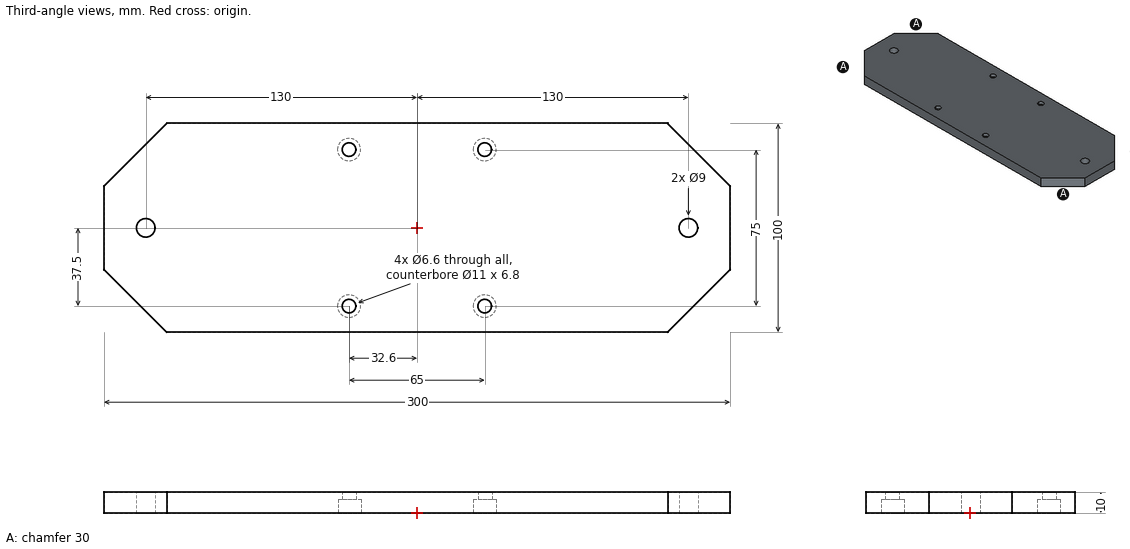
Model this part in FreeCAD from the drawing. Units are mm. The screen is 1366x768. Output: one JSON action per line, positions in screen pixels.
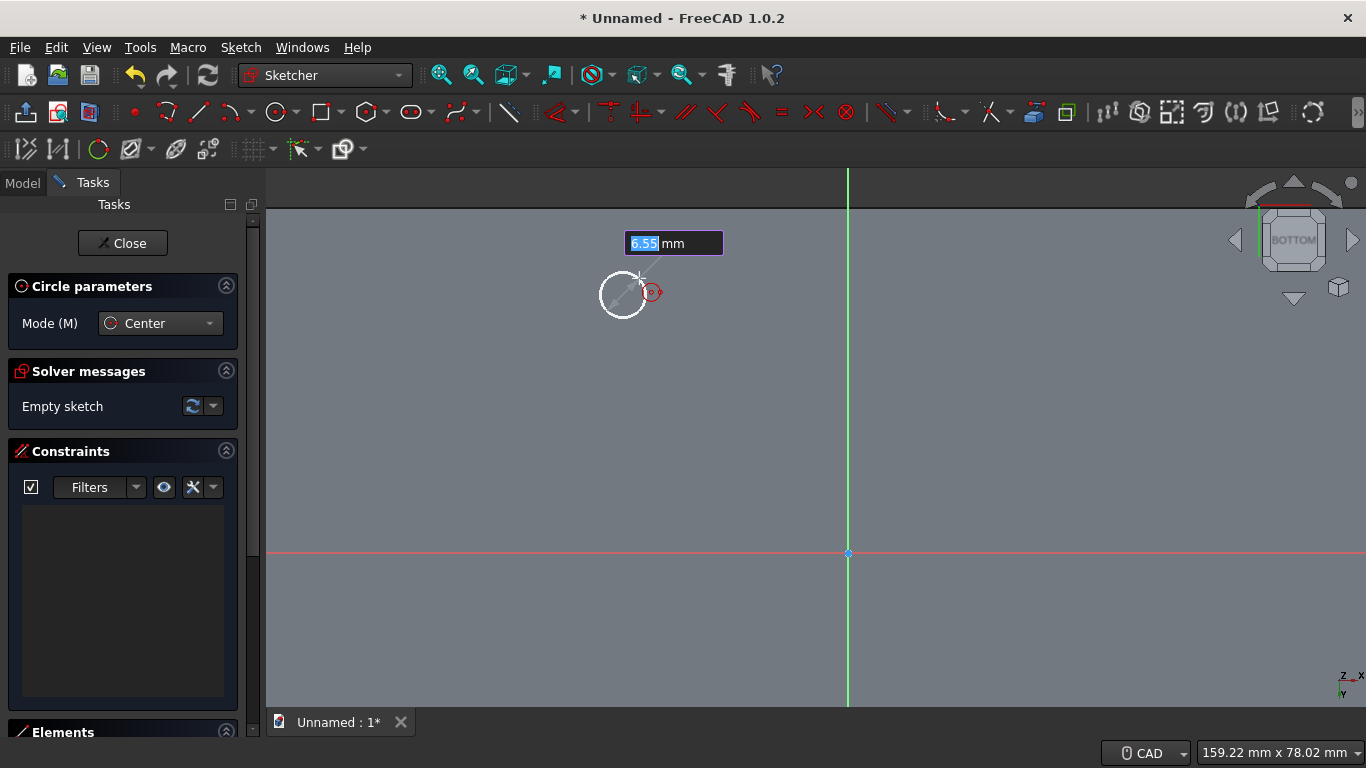
{"action": "type", "text": "6.6"}
{"action": "key", "text": "Return"}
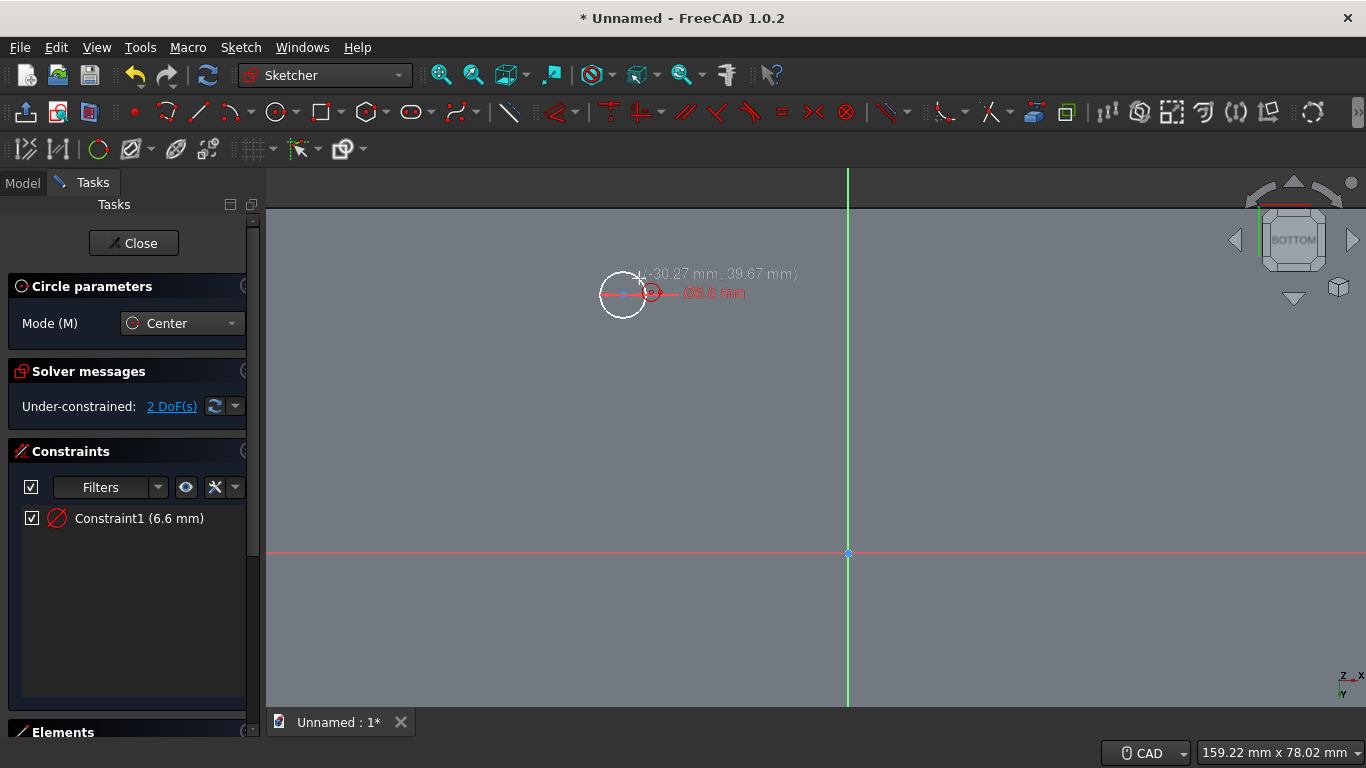
{"action": "left_click", "coordinate": [1072, 294]}
{"action": "mouse_move", "coordinate": [1088, 278]}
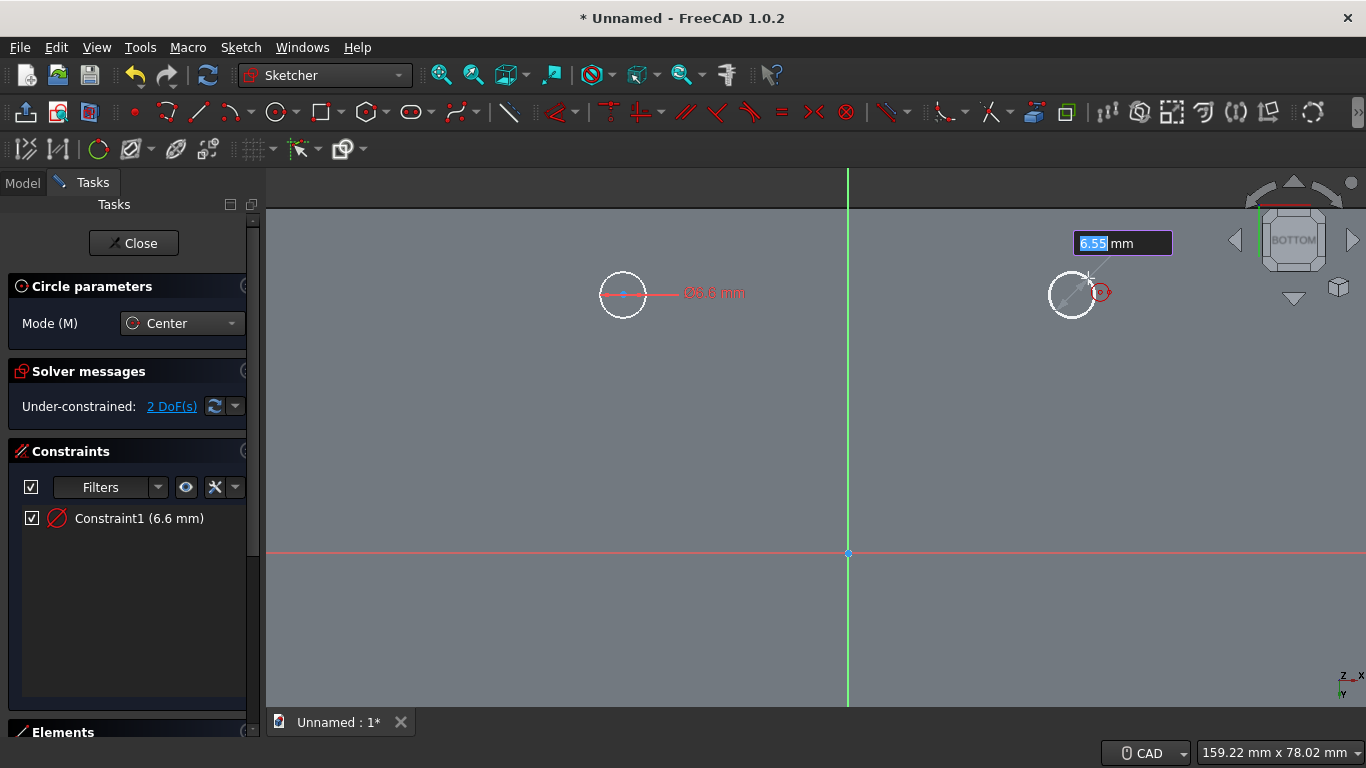
{"action": "type", "text": "6.6"}
{"action": "key", "text": "Return"}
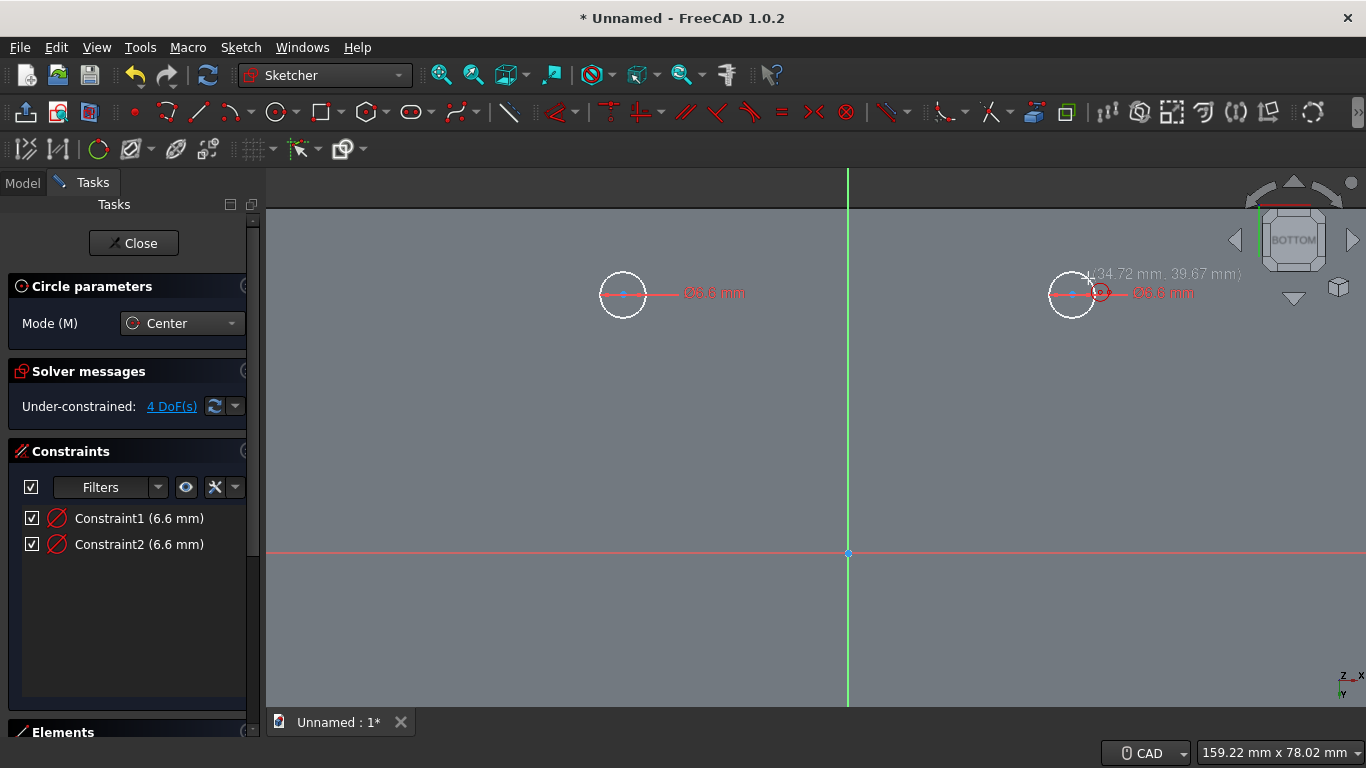
{"action": "scroll", "coordinate": [626, 297], "scroll_direction": "down", "scroll_amount": 3}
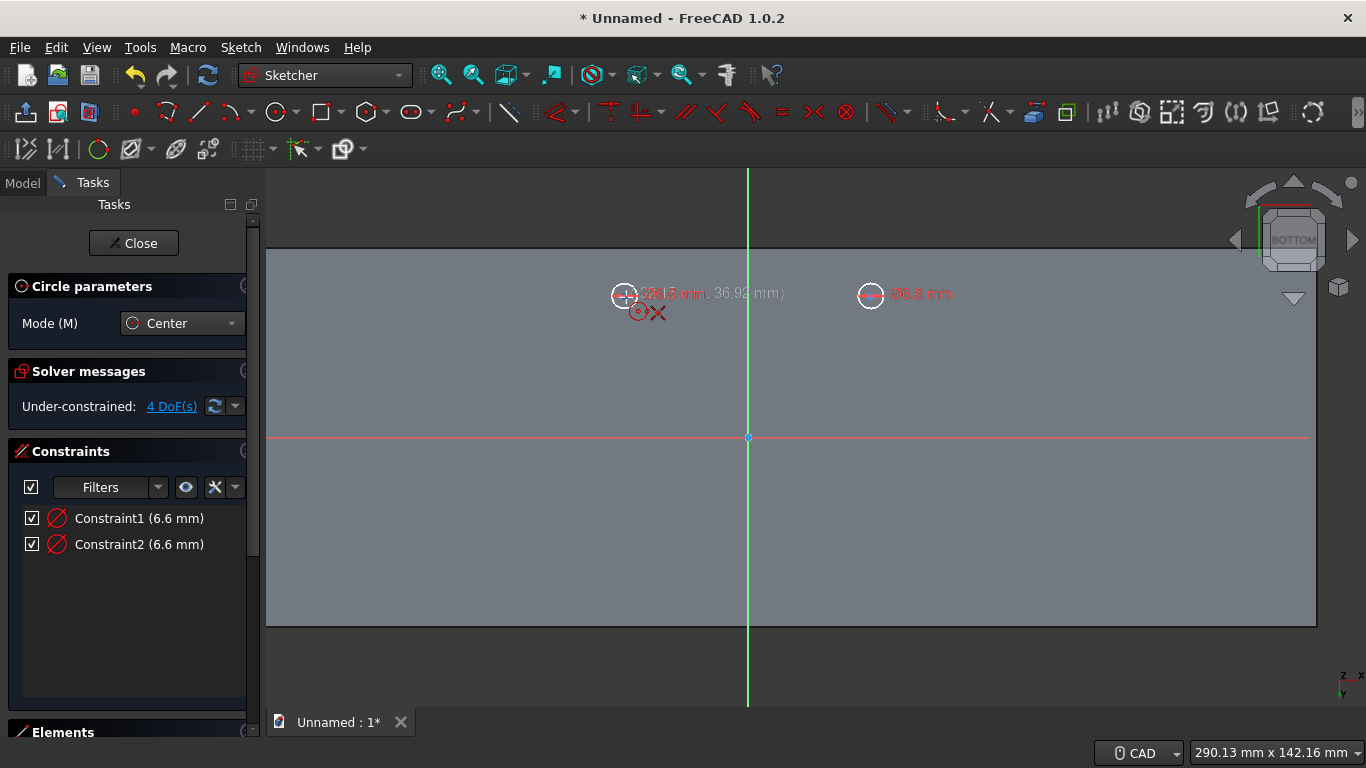
{"action": "scroll", "coordinate": [871, 580], "scroll_direction": "up", "scroll_amount": 3}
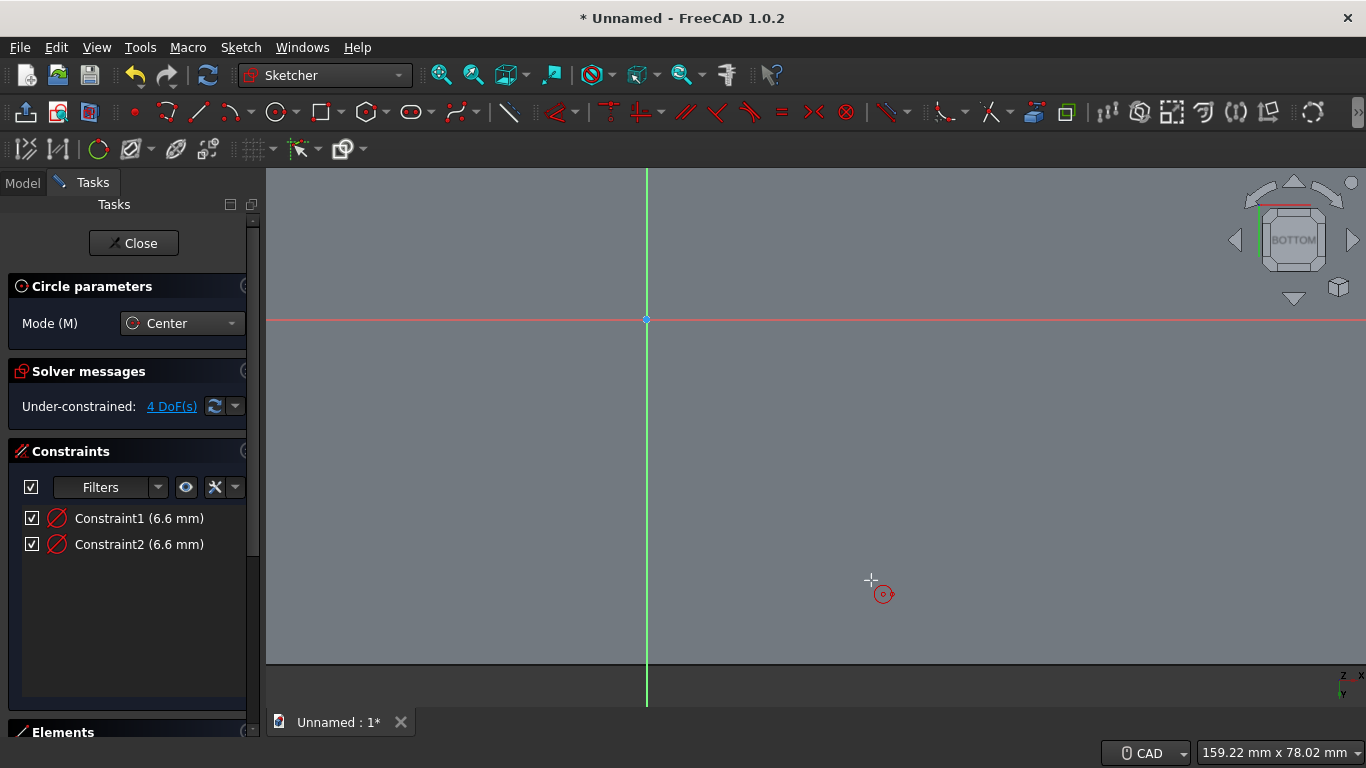
{"action": "left_click", "coordinate": [870, 579]}
{"action": "mouse_move", "coordinate": [886, 563]}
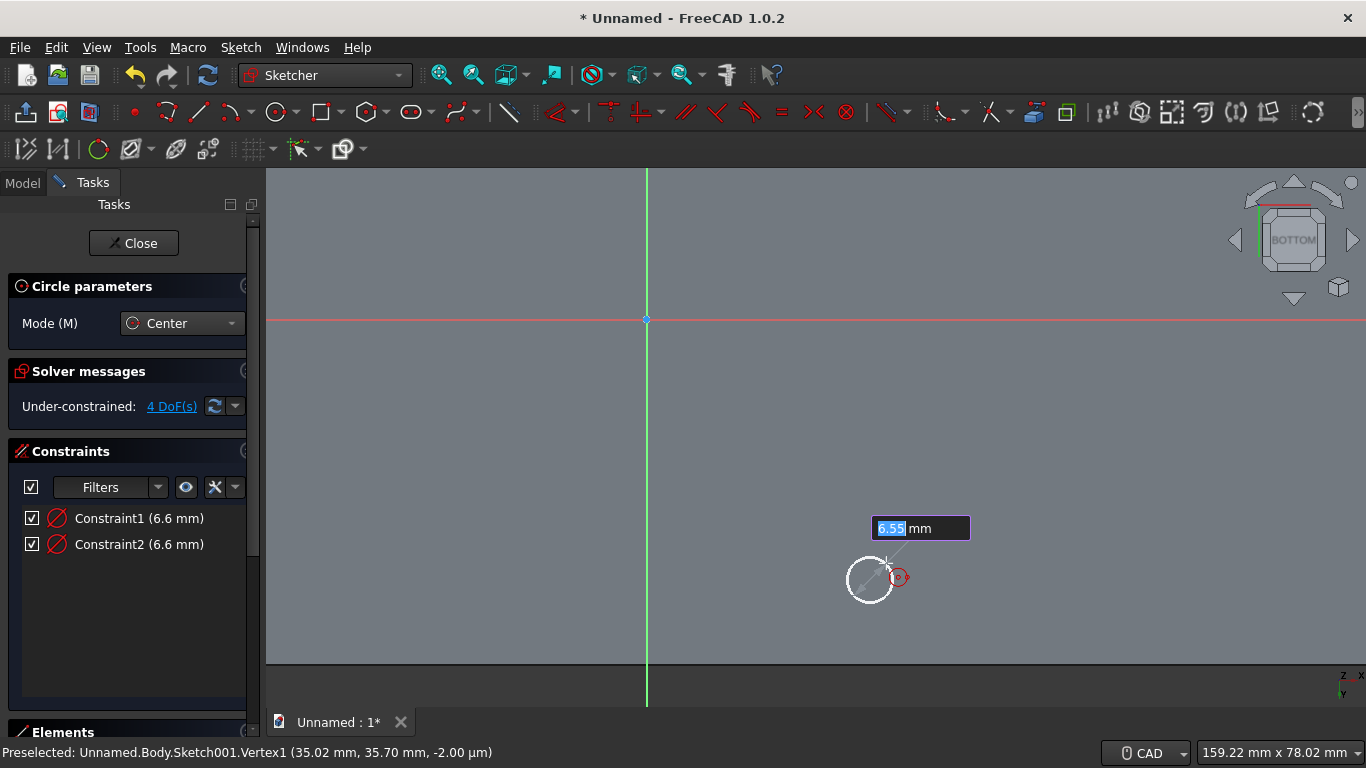
{"action": "type", "text": "6.6"}
{"action": "key", "text": "Return"}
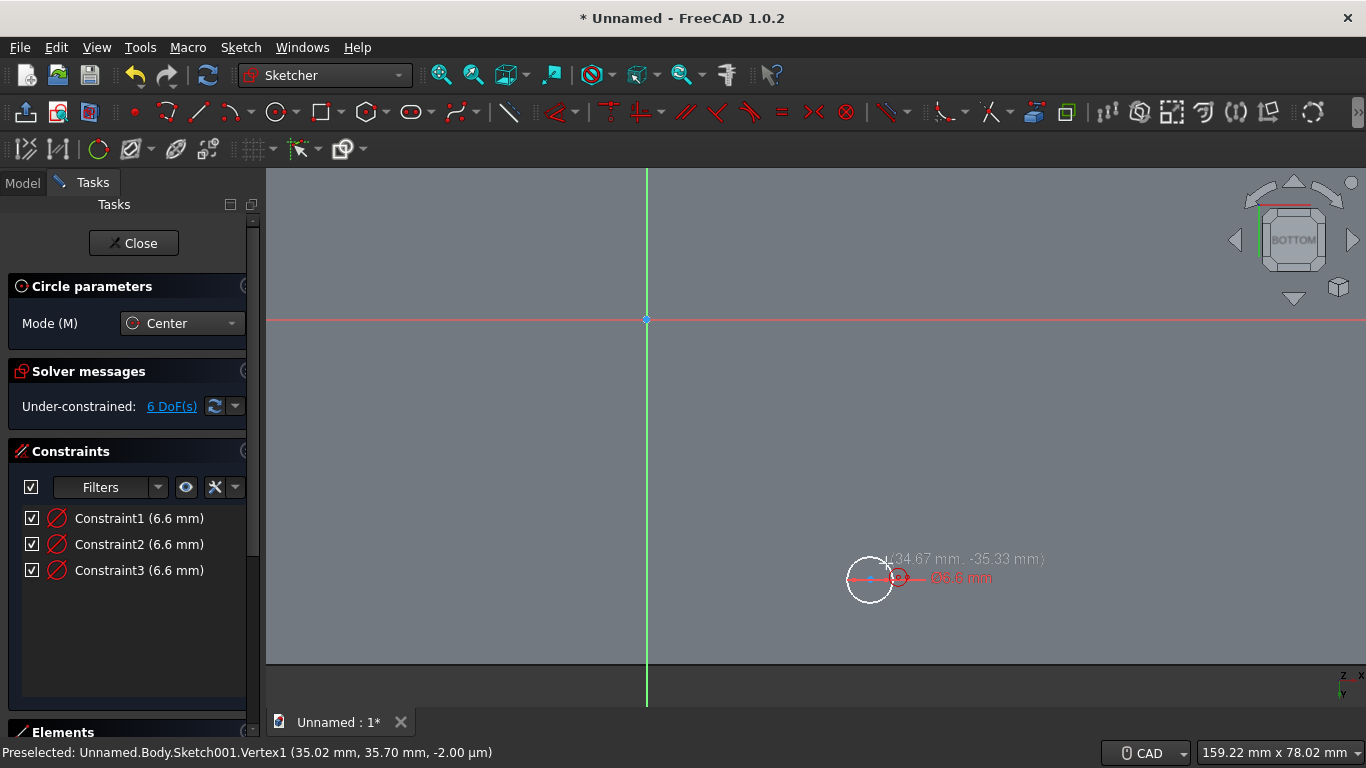
{"action": "left_click", "coordinate": [421, 579]}
{"action": "mouse_move", "coordinate": [437, 563]}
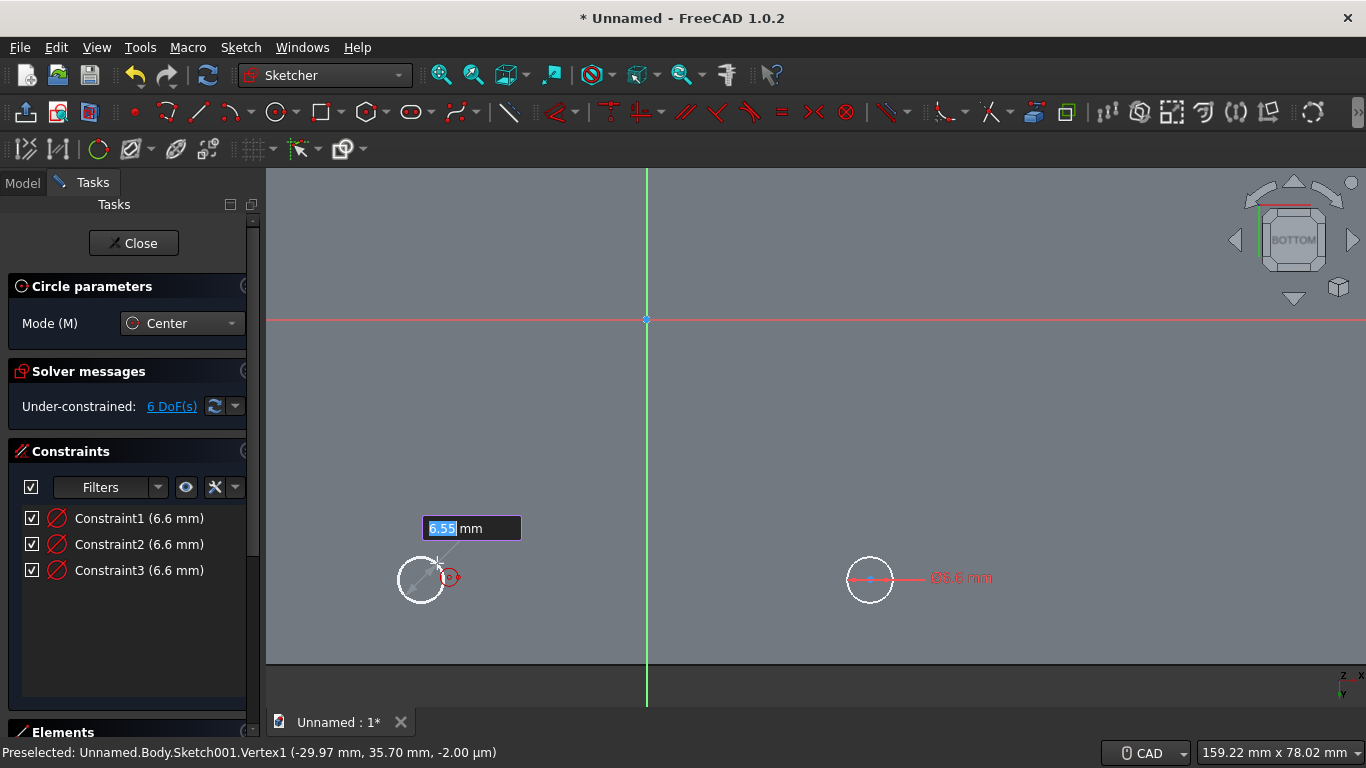
{"action": "type", "text": "6.6"}
{"action": "key", "text": "Return"}
{"action": "key", "text": "Escape"}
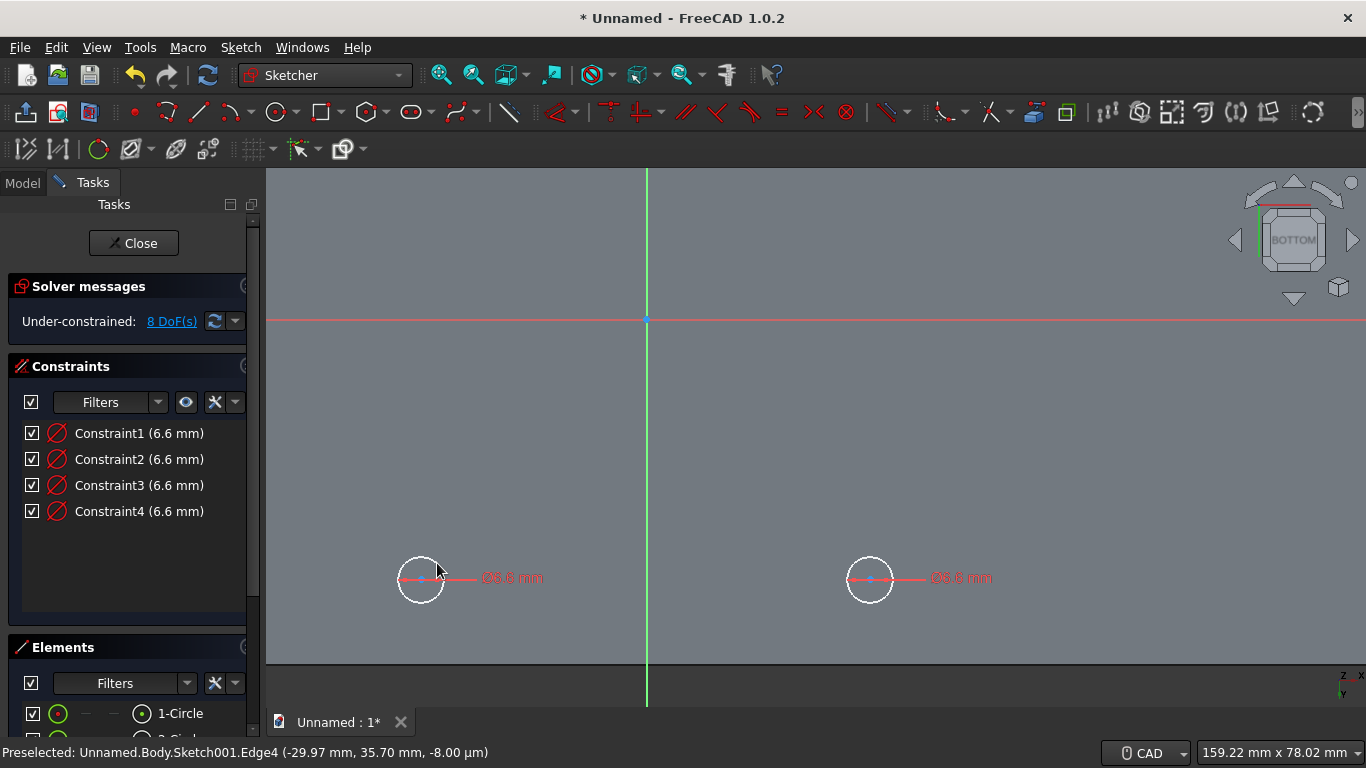
{"action": "scroll", "coordinate": [871, 580], "scroll_direction": "down", "scroll_amount": 3}